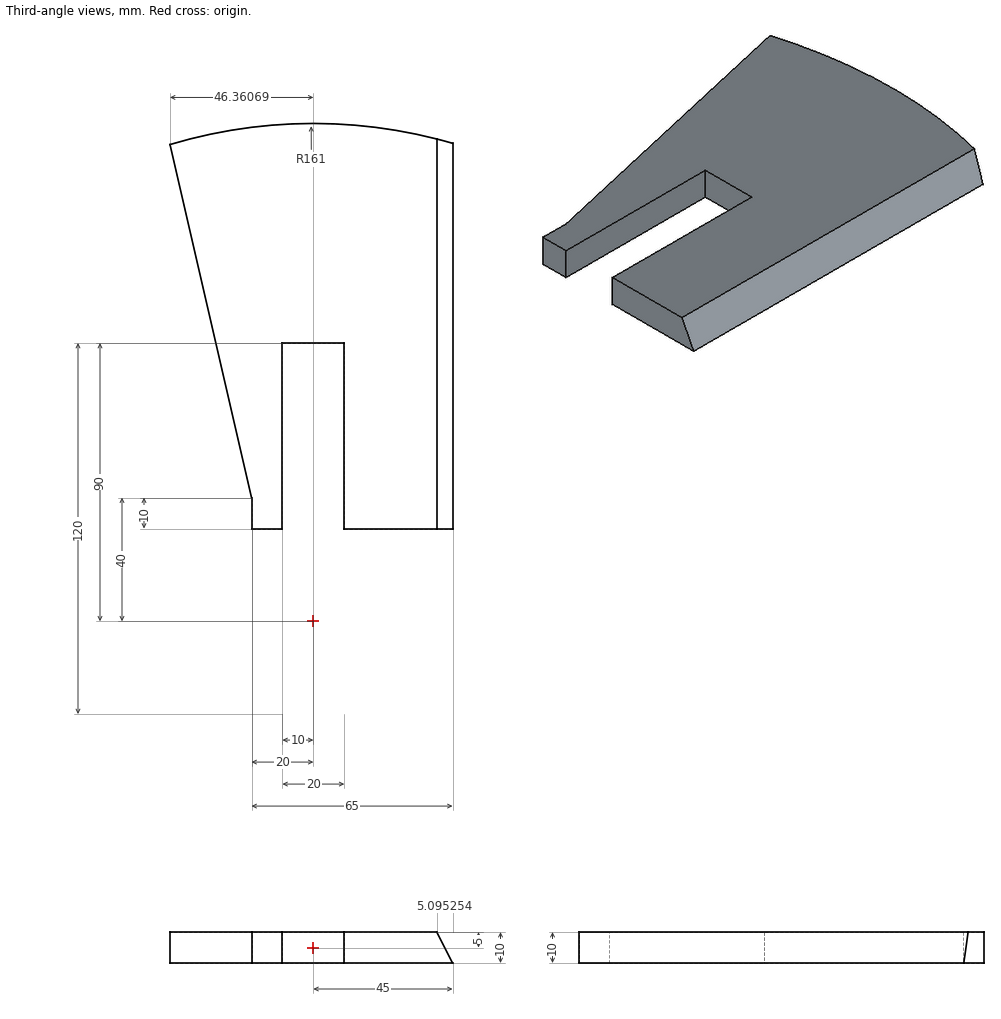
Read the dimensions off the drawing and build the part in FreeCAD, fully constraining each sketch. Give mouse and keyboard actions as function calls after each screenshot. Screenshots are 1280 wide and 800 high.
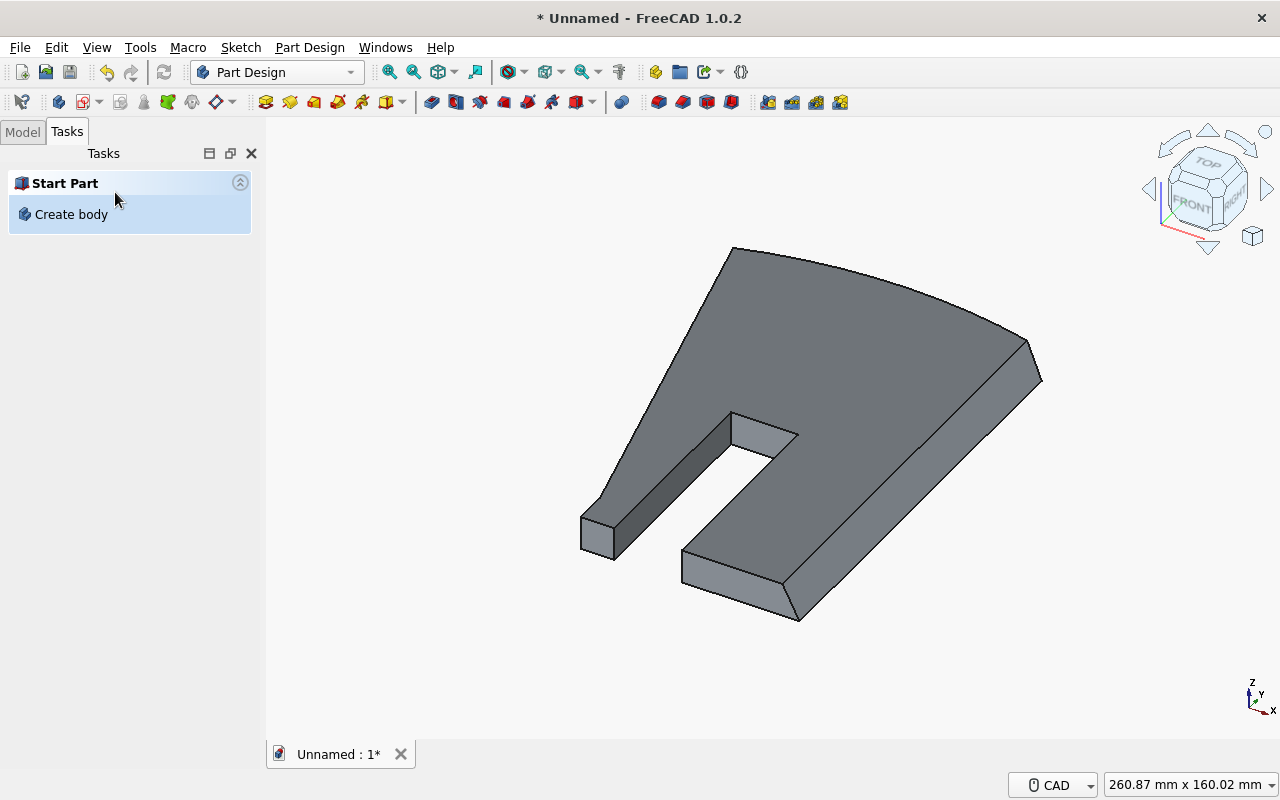
key(0)